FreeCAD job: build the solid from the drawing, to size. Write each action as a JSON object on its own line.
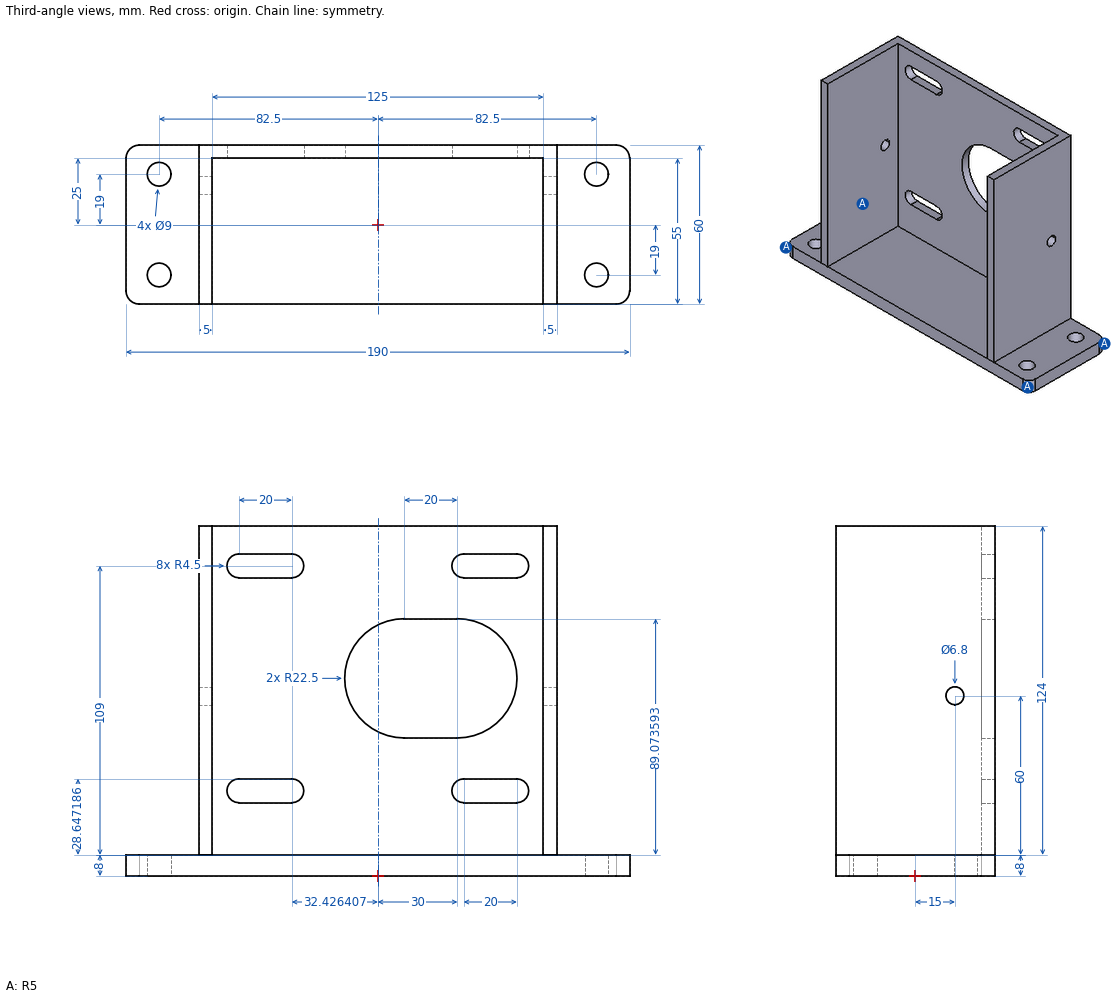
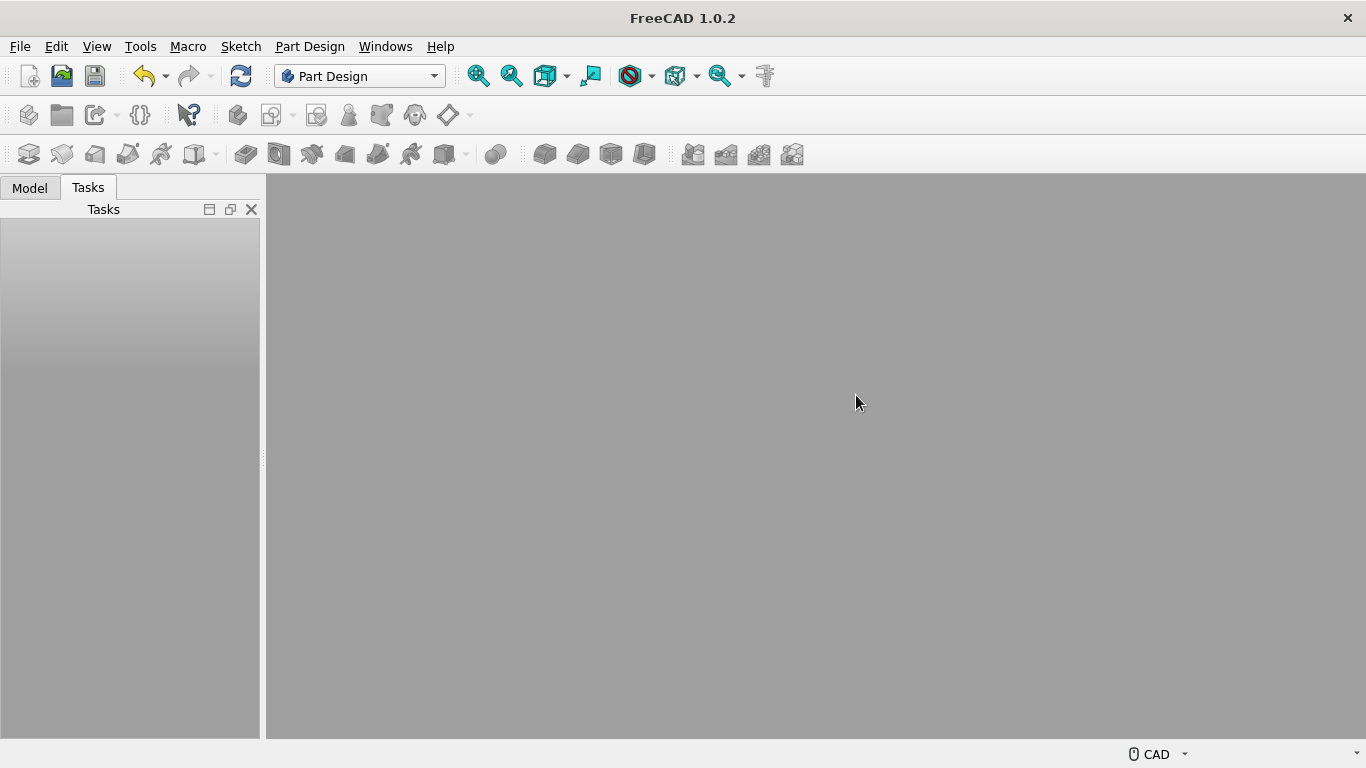
{"action": "left_click", "coordinate": [29, 76]}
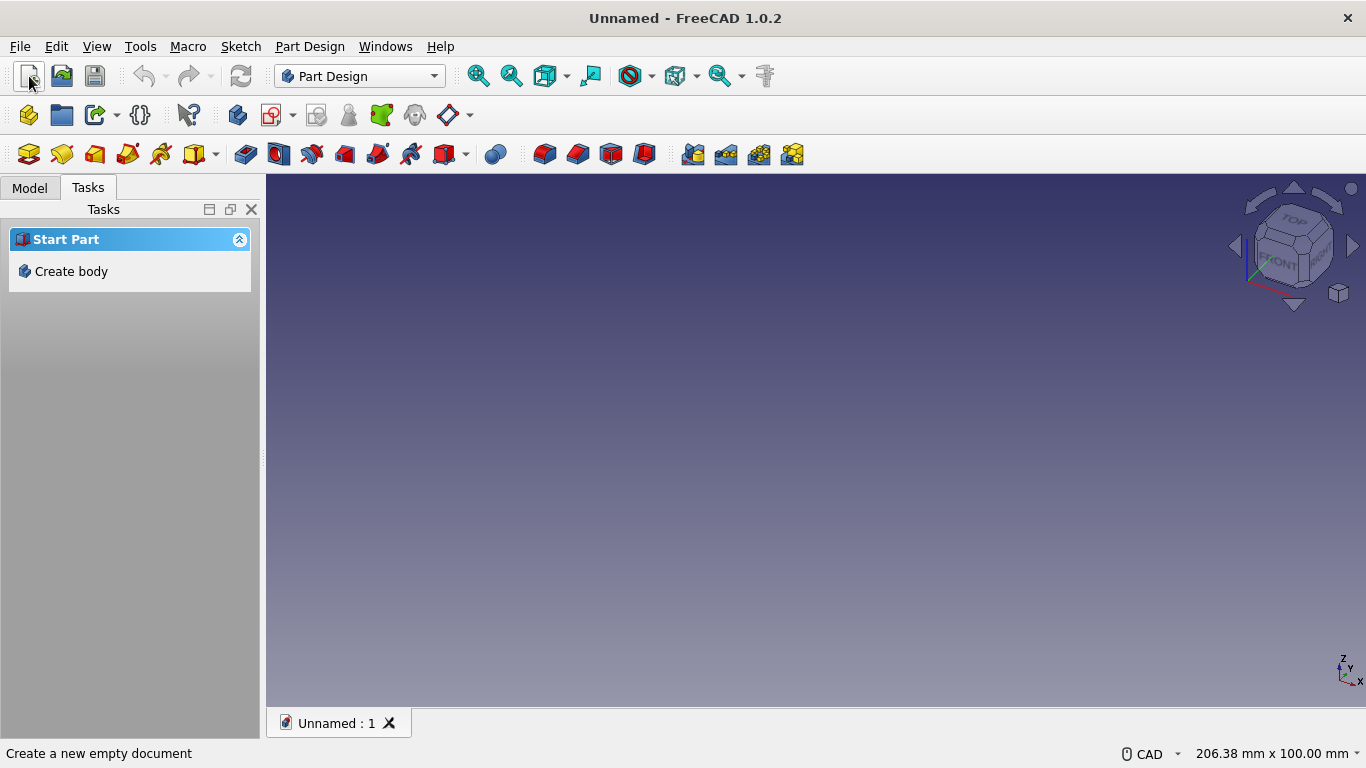
{"action": "left_click", "coordinate": [270, 116]}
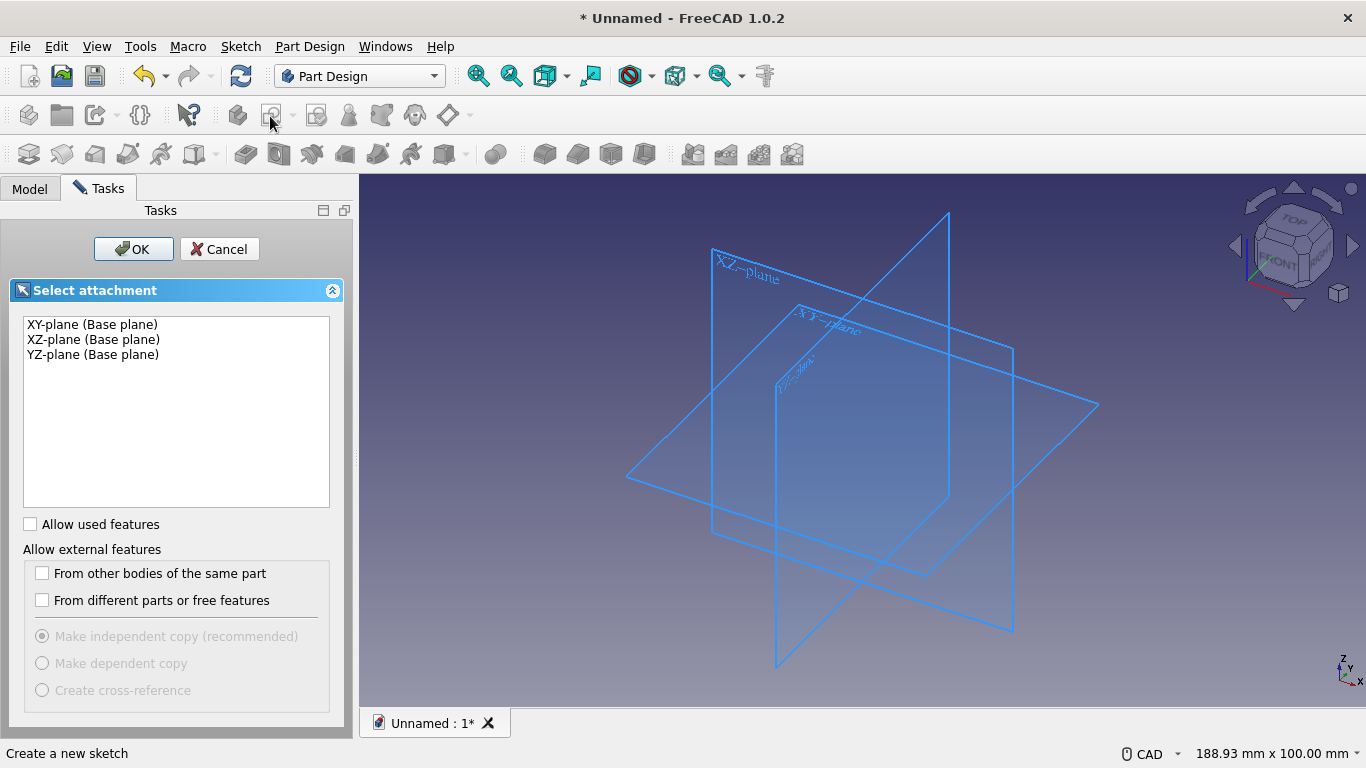
{"action": "left_click", "coordinate": [84, 324]}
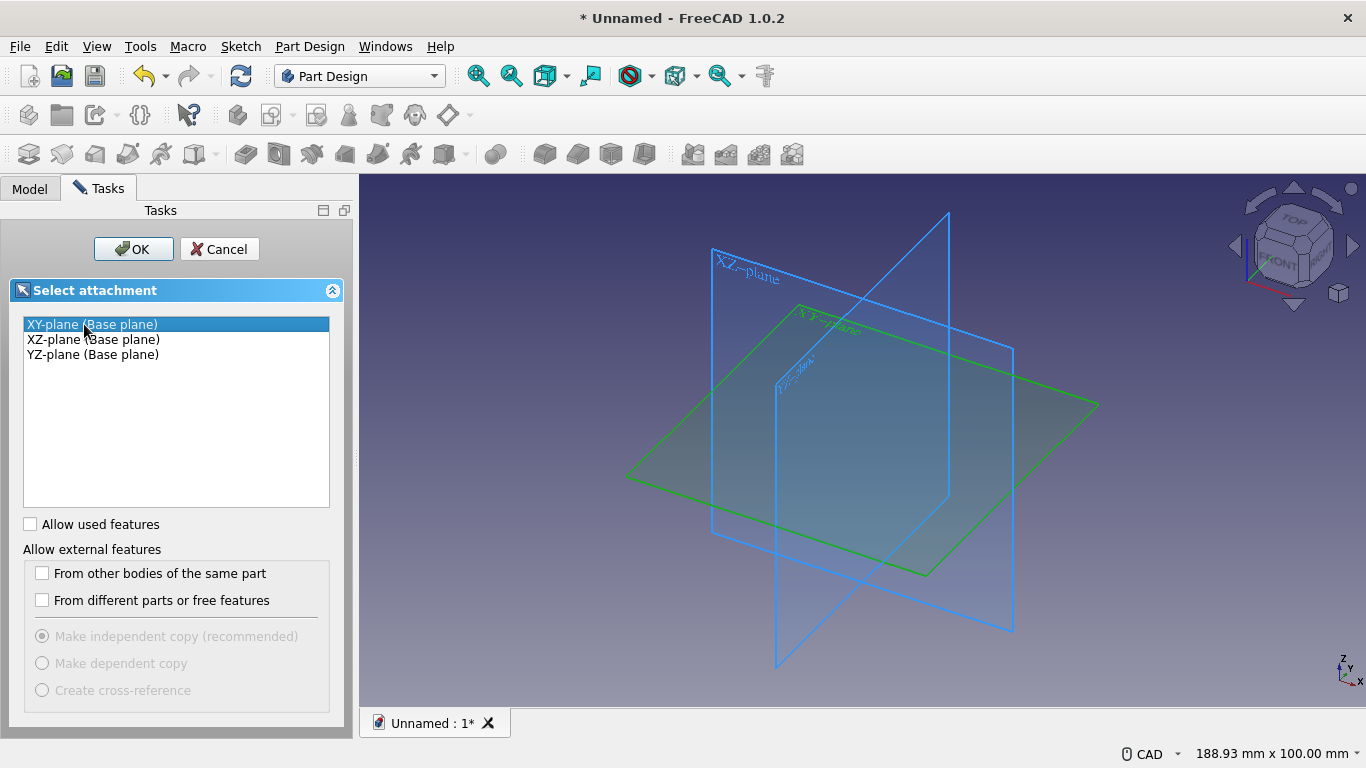
{"action": "left_click", "coordinate": [134, 249]}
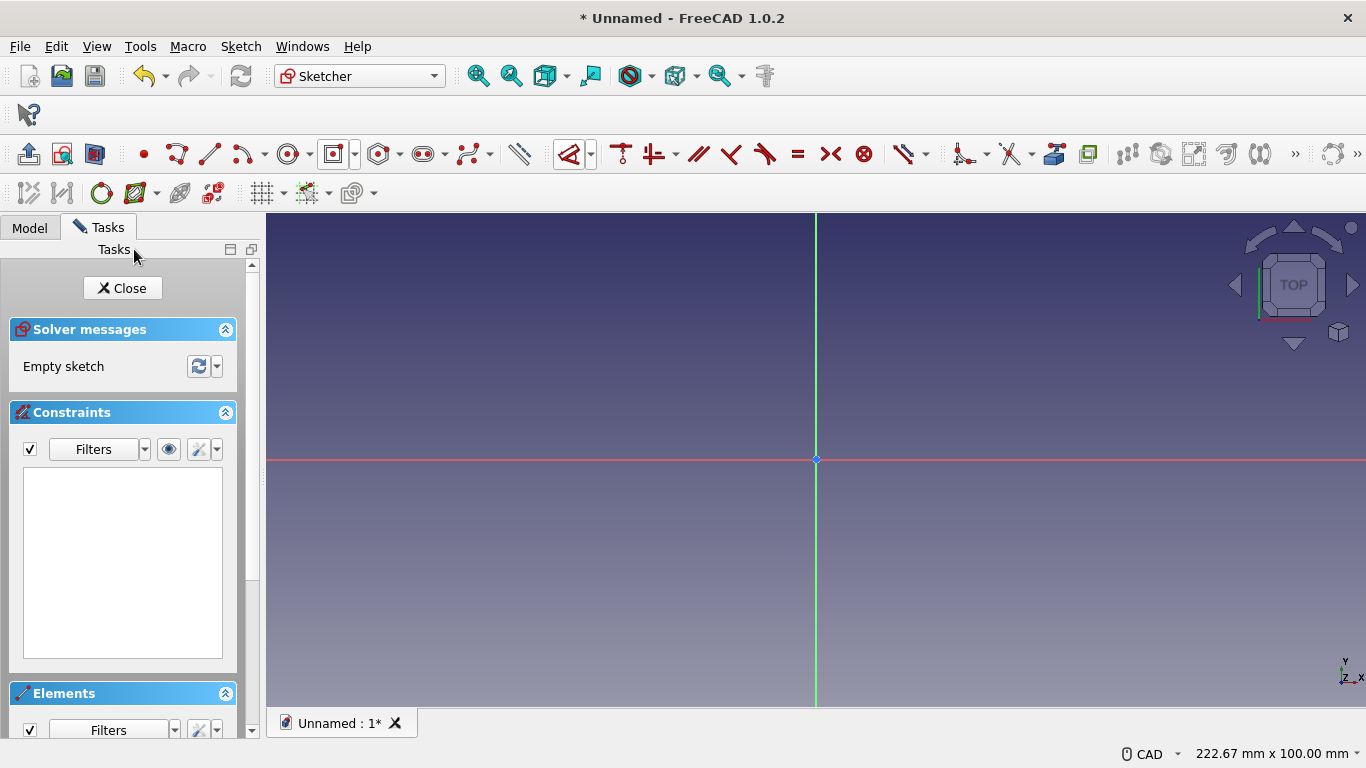
{"action": "scroll", "coordinate": [608, 460], "scroll_direction": "down", "scroll_amount": 2}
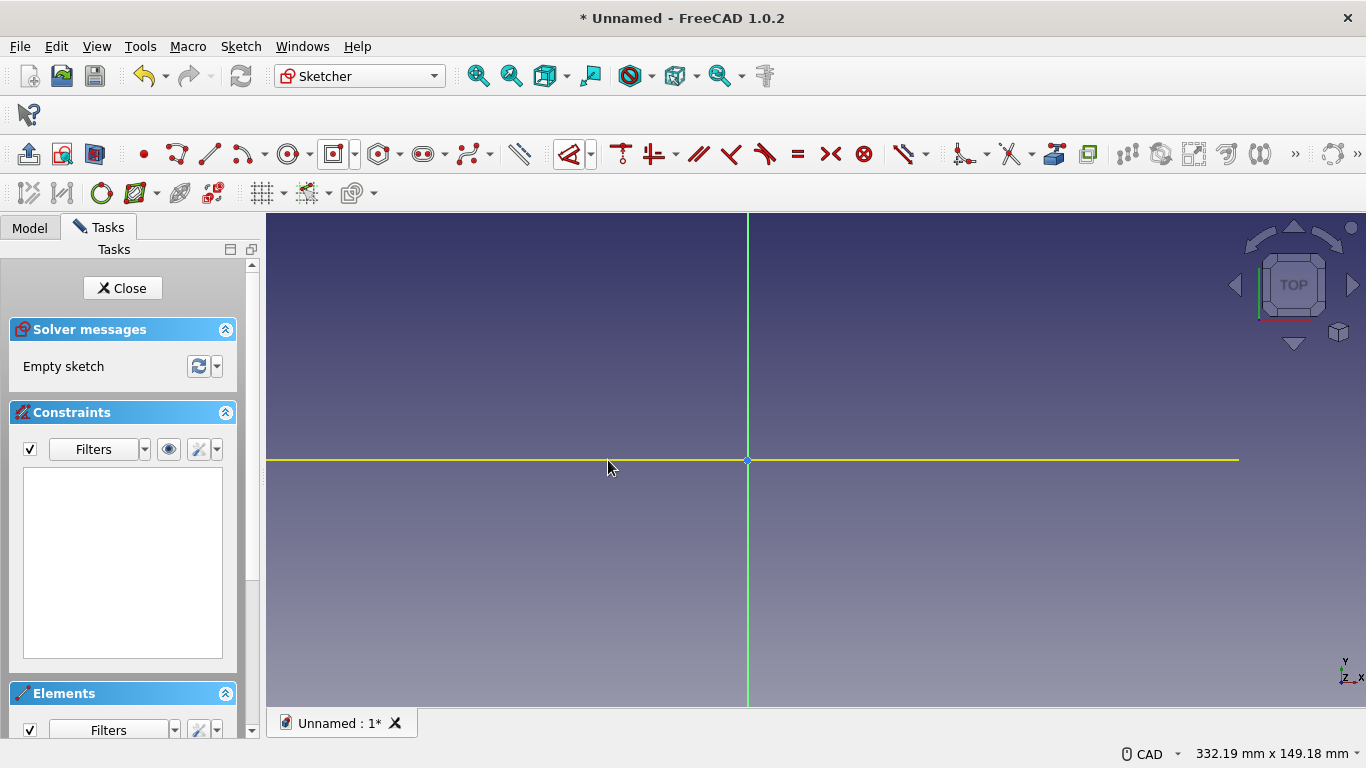
{"action": "left_click", "coordinate": [332, 154]}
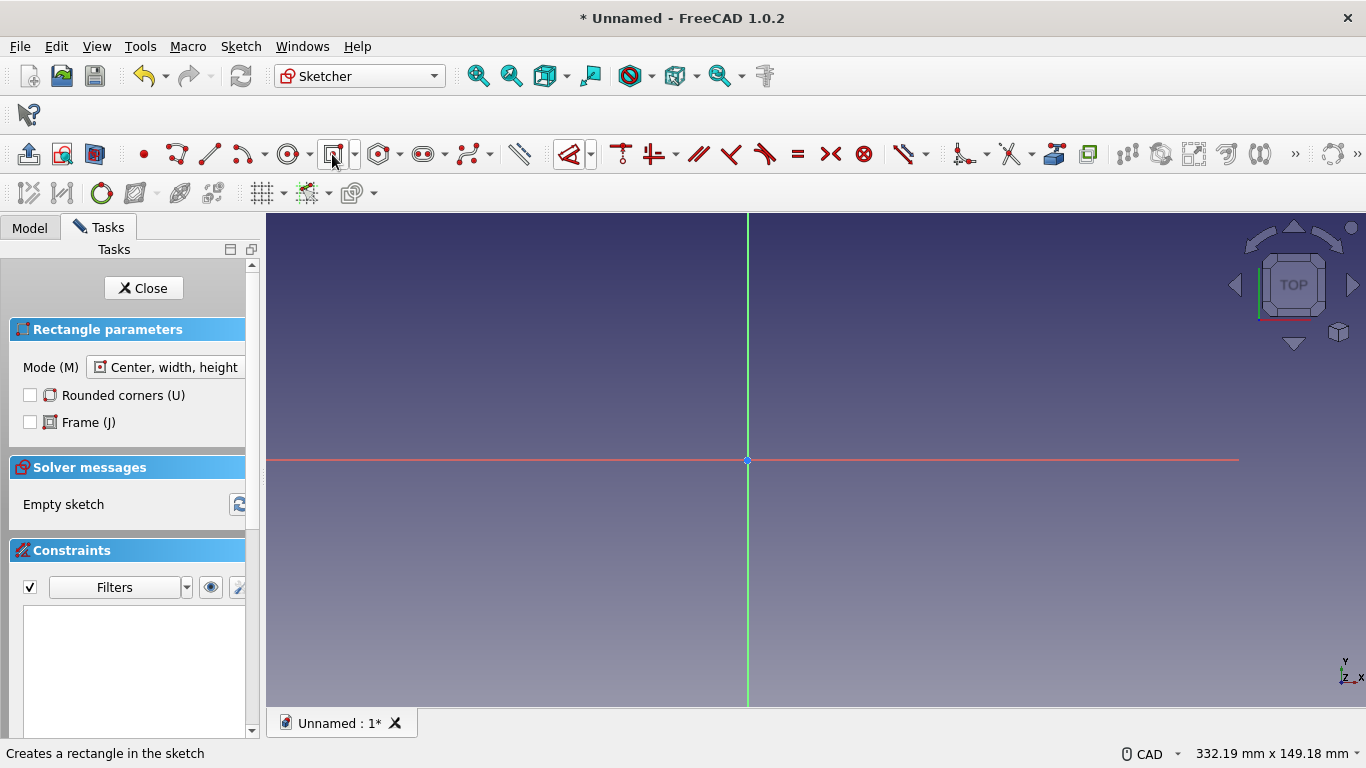
{"action": "left_click", "coordinate": [748, 460]}
{"action": "mouse_move", "coordinate": [1062, 361]}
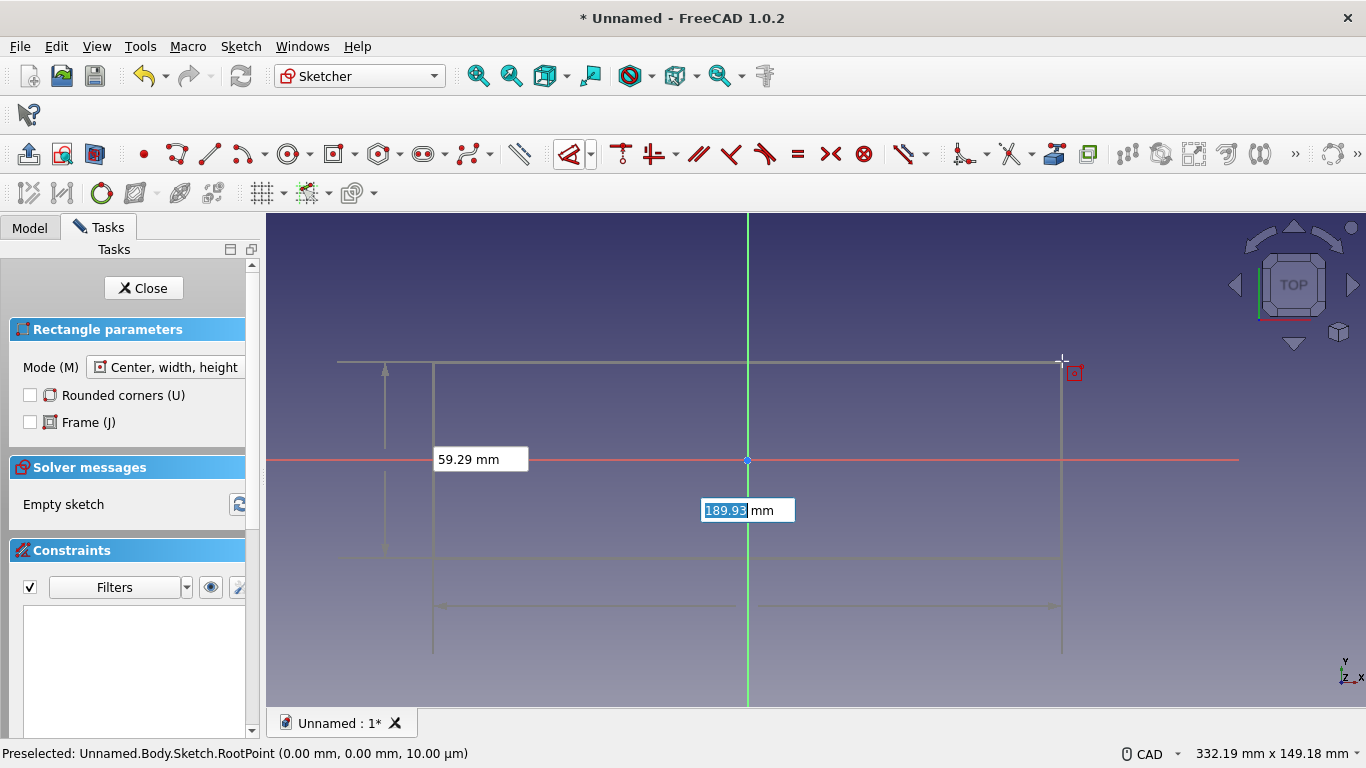
{"action": "type", "text": "190"}
{"action": "key", "text": "Tab"}
{"action": "type", "text": "60"}
{"action": "key", "text": "Return"}
{"action": "key", "text": "Escape"}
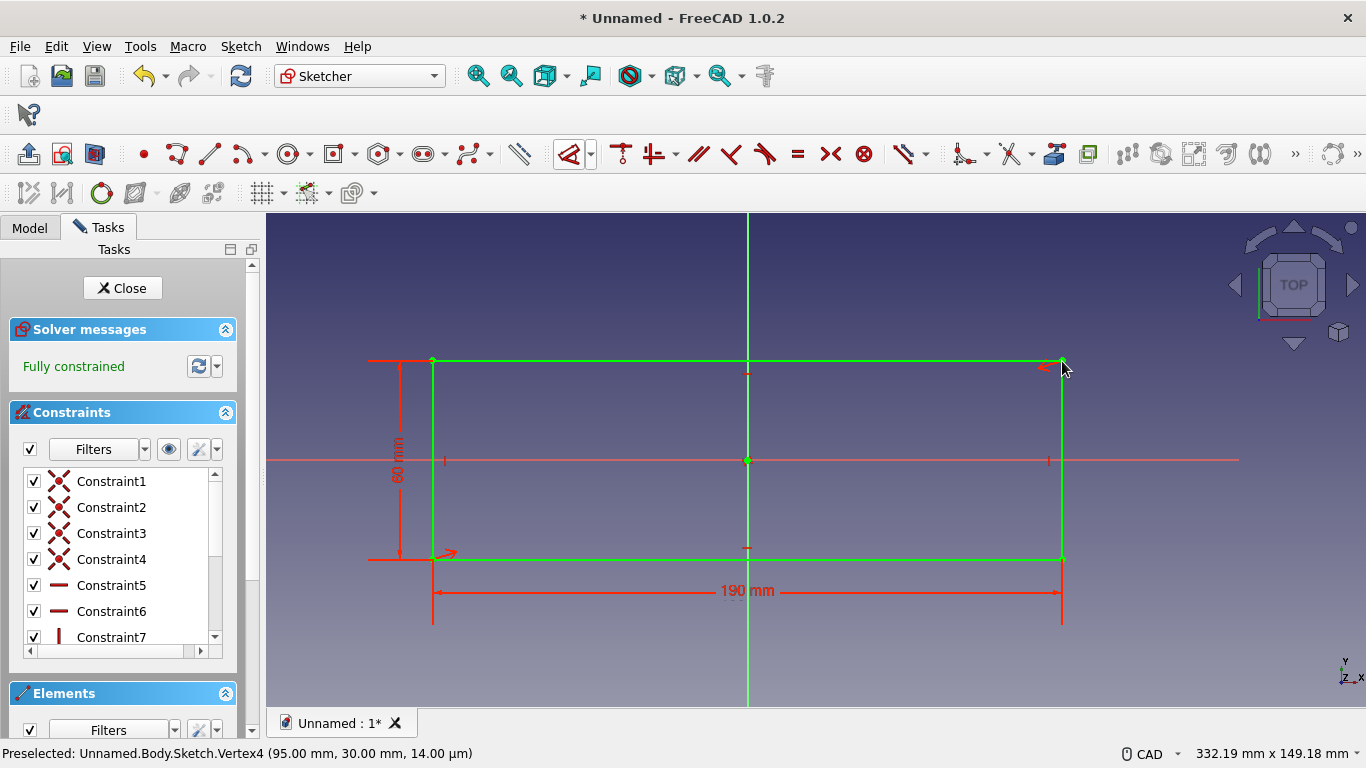
{"action": "left_click", "coordinate": [123, 288]}